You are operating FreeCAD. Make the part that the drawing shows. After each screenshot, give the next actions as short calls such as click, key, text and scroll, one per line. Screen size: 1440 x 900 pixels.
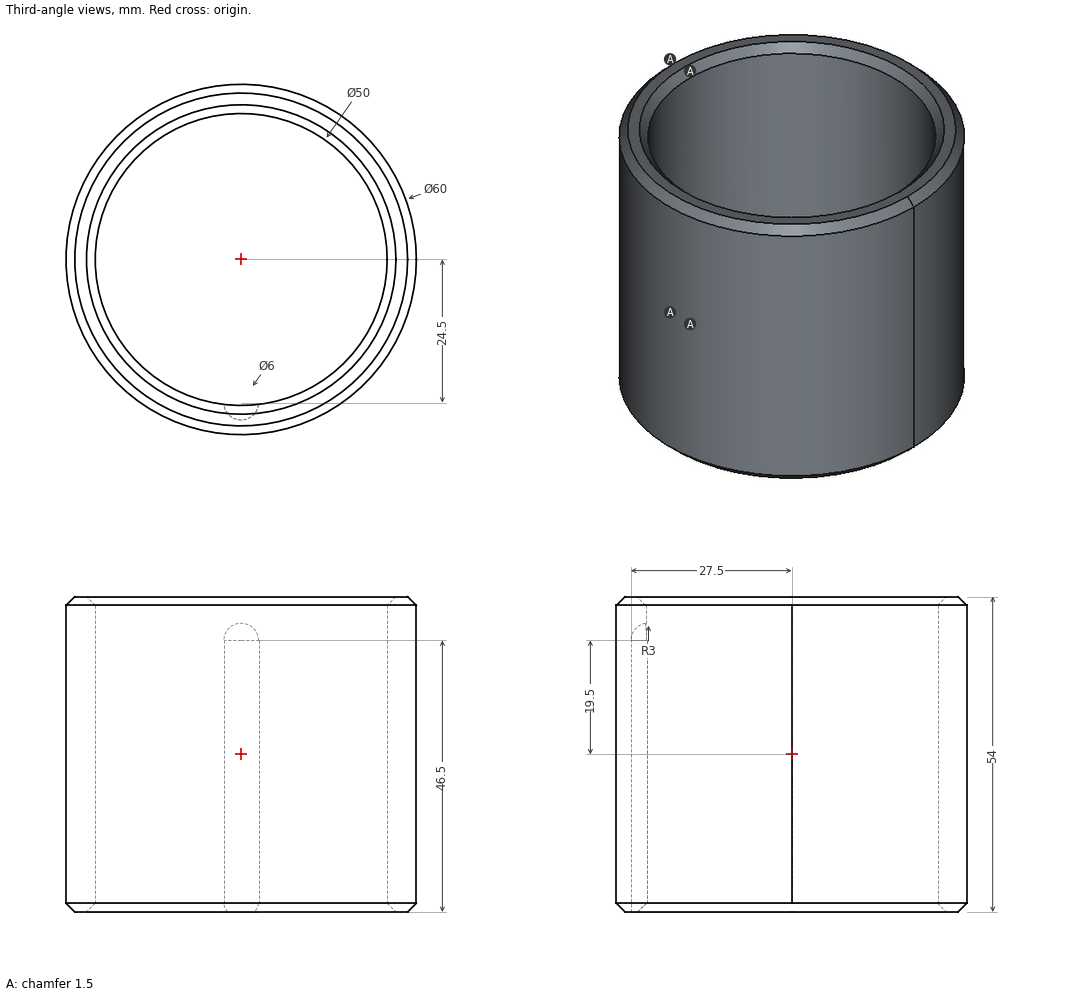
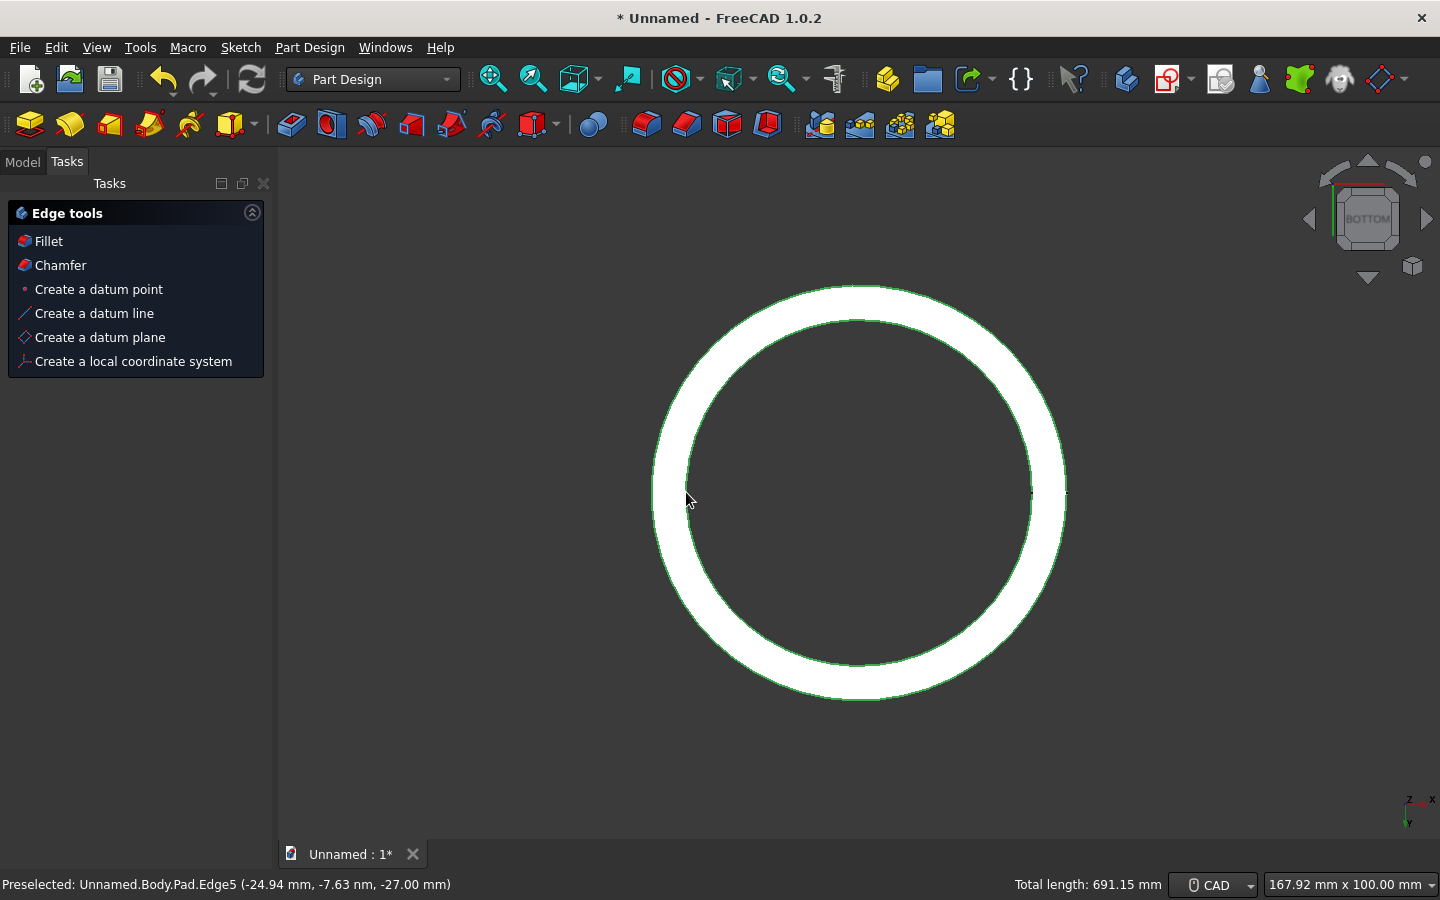
click(688, 124)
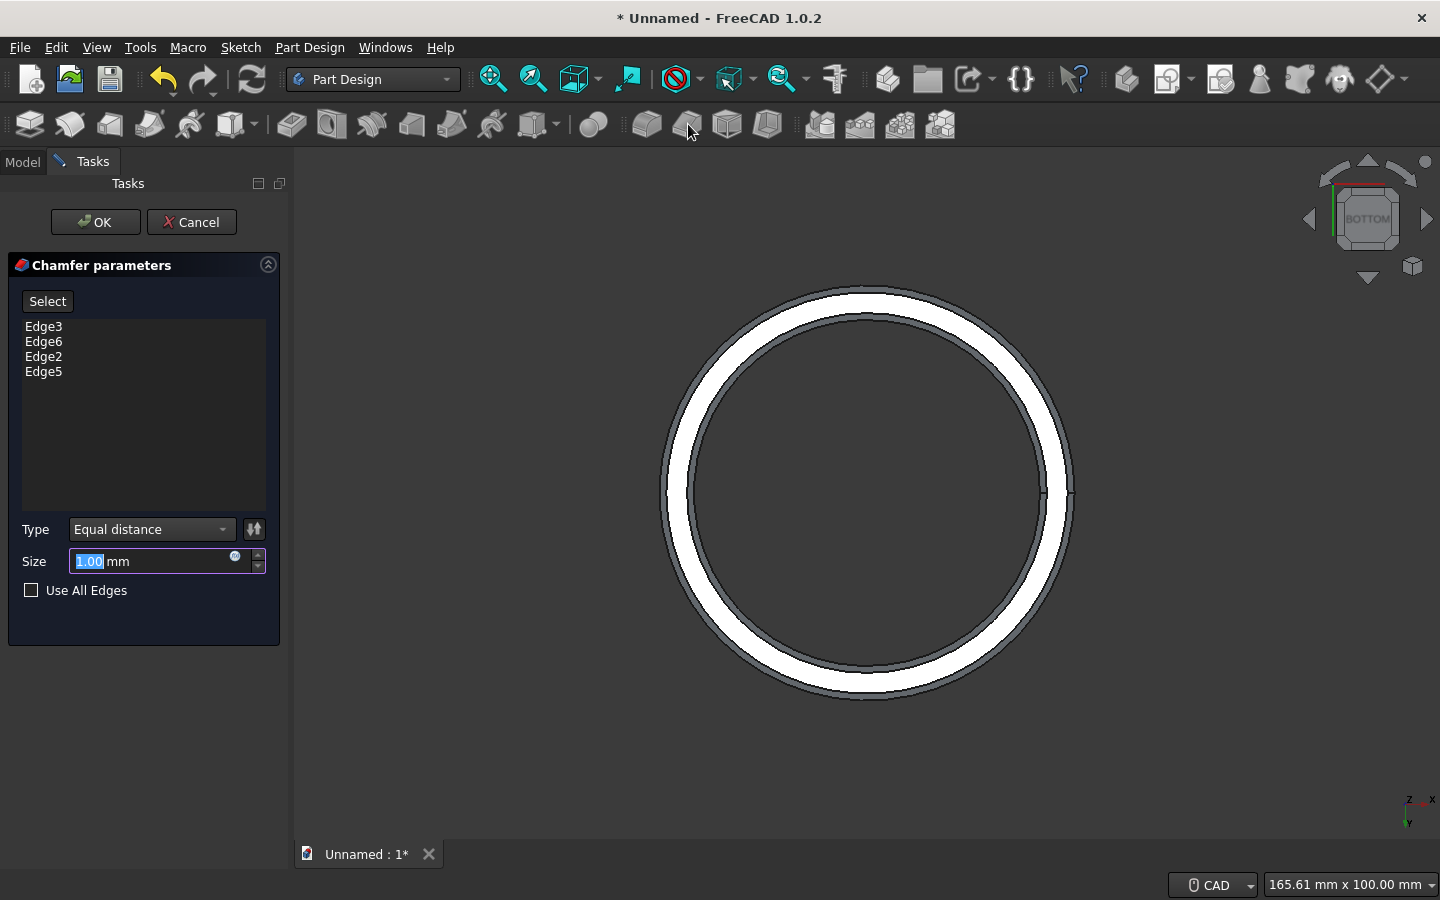
text(1.5)
key(Tab)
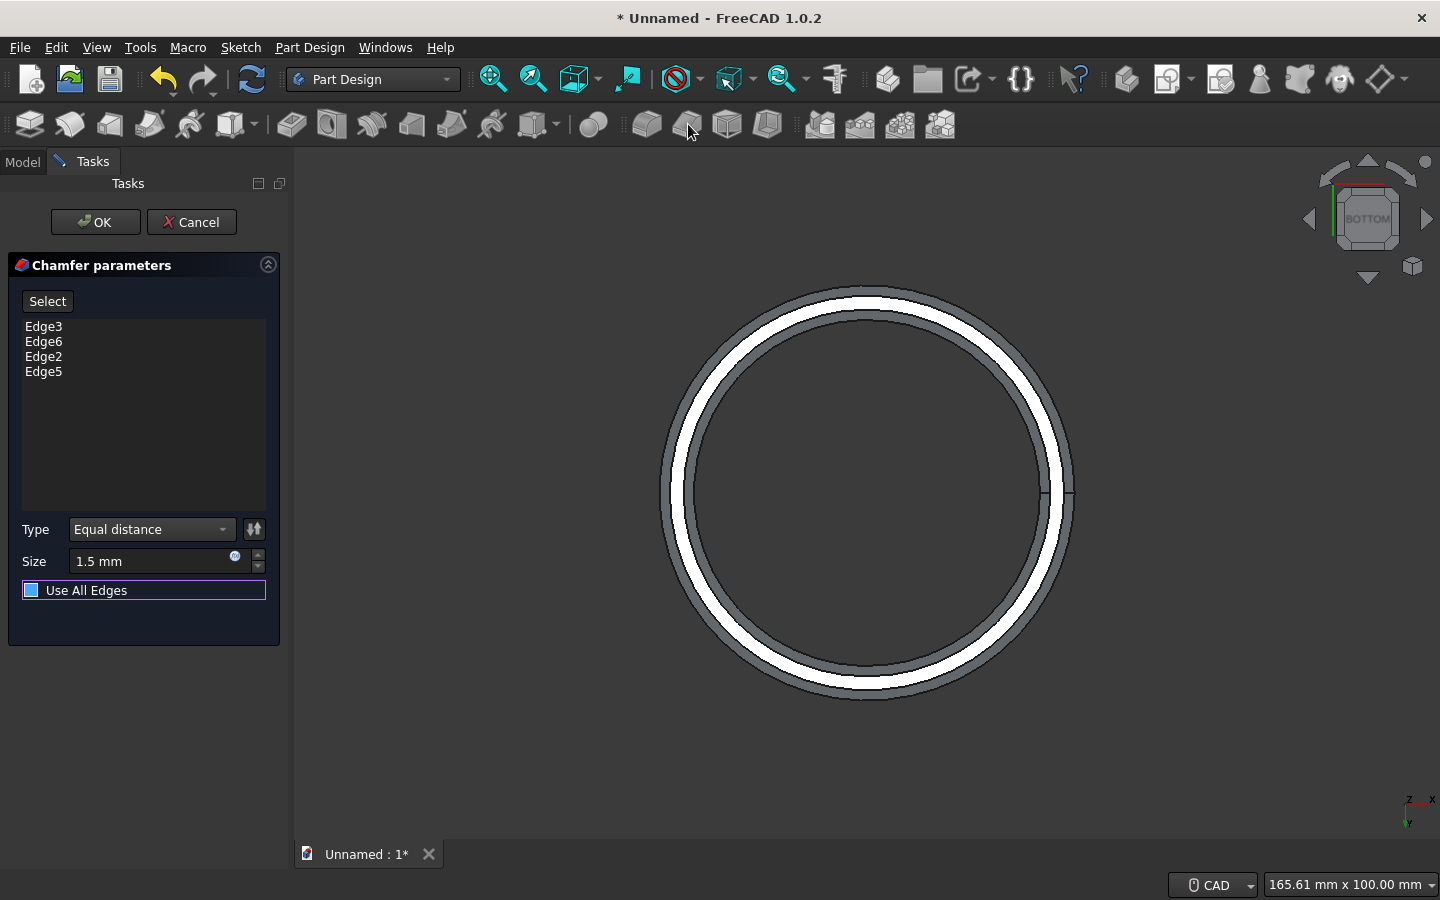
click(96, 222)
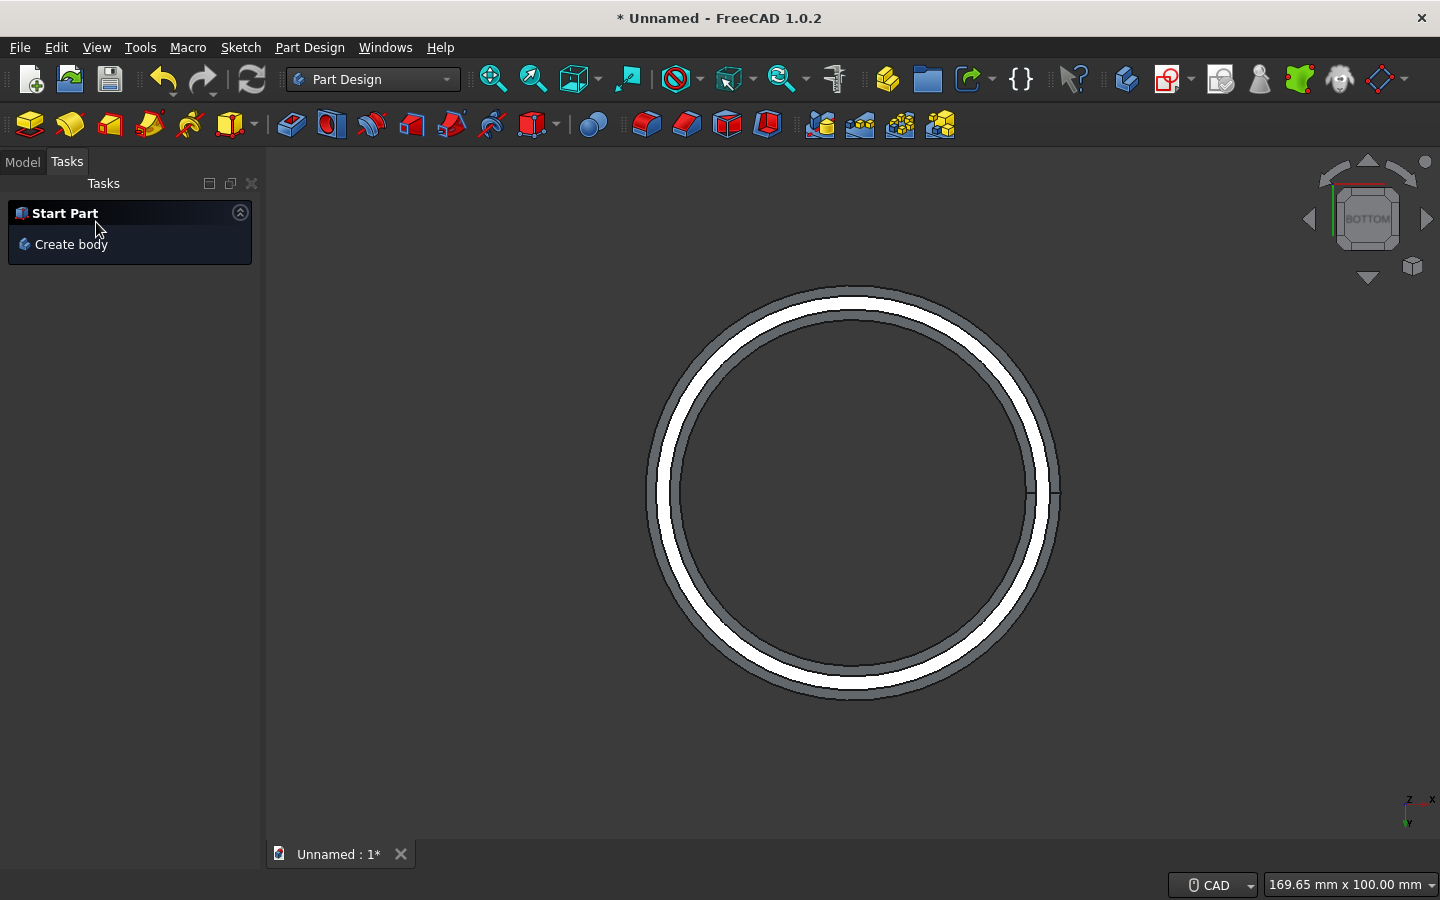
click(1168, 80)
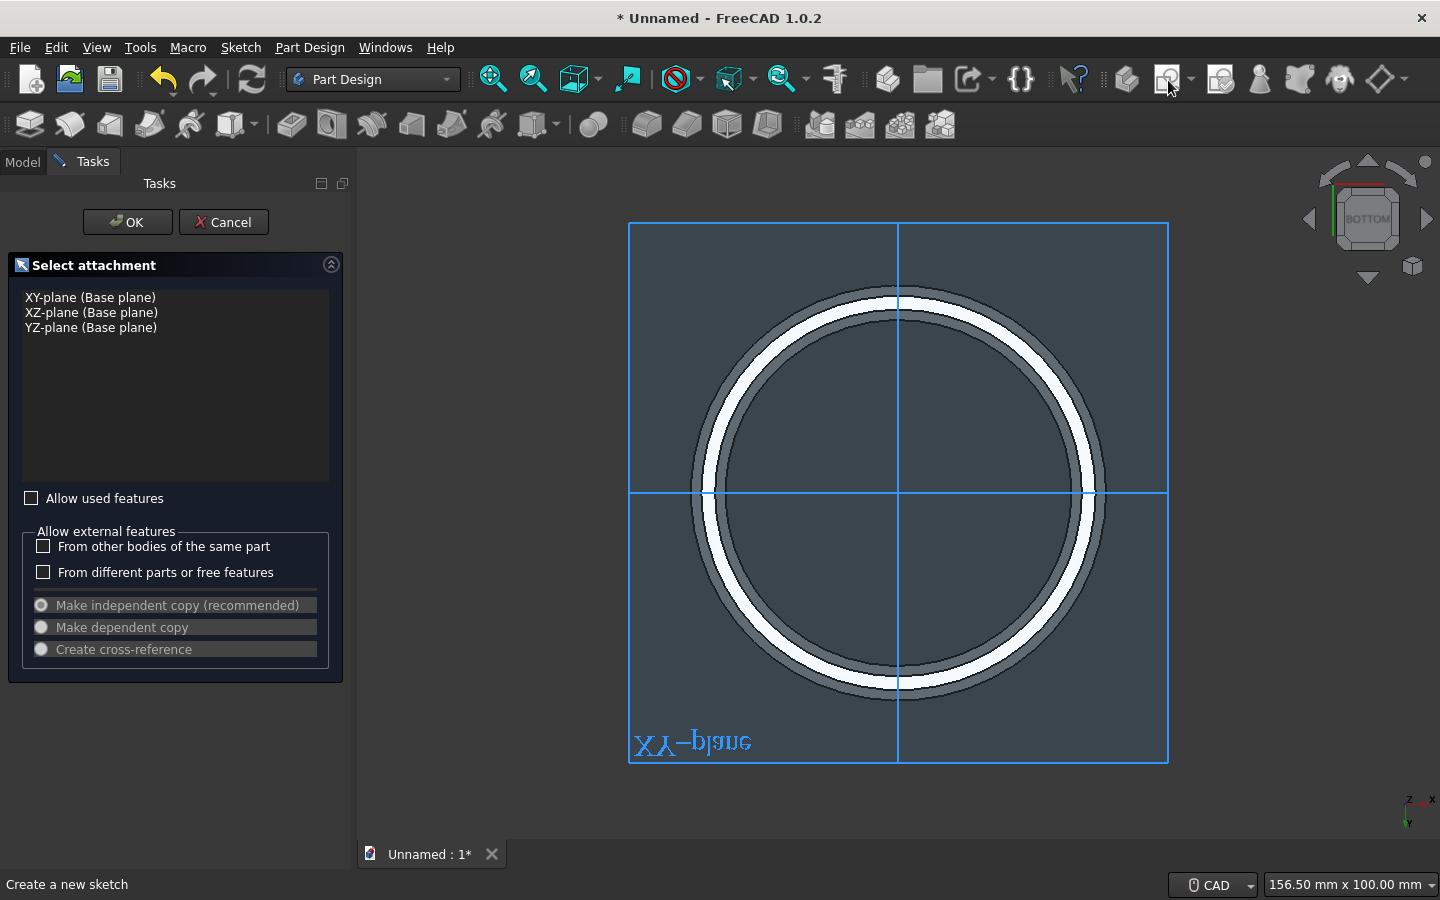
click(82, 328)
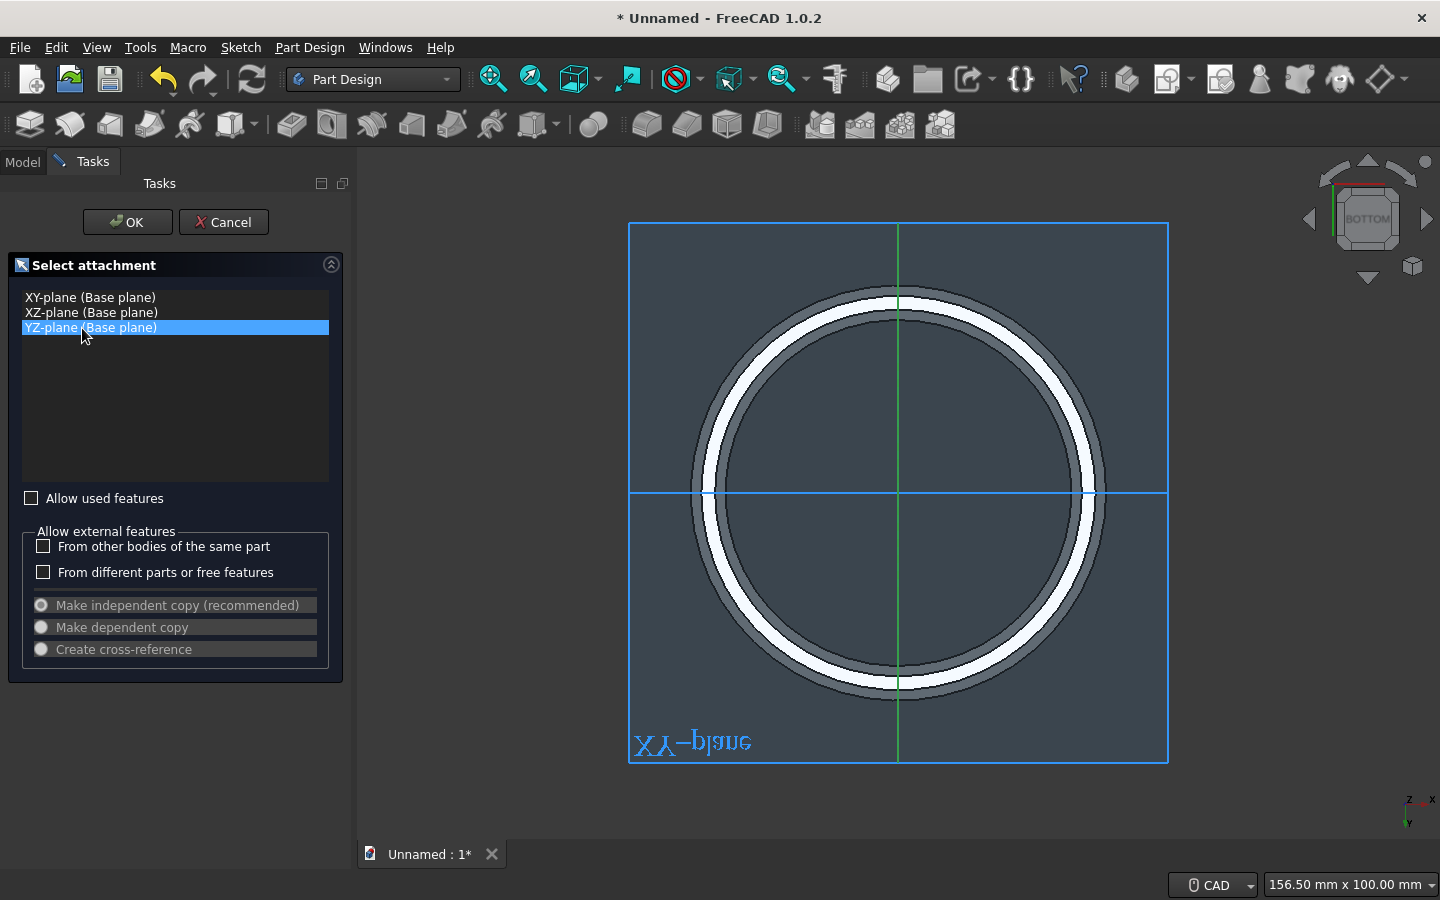
click(128, 222)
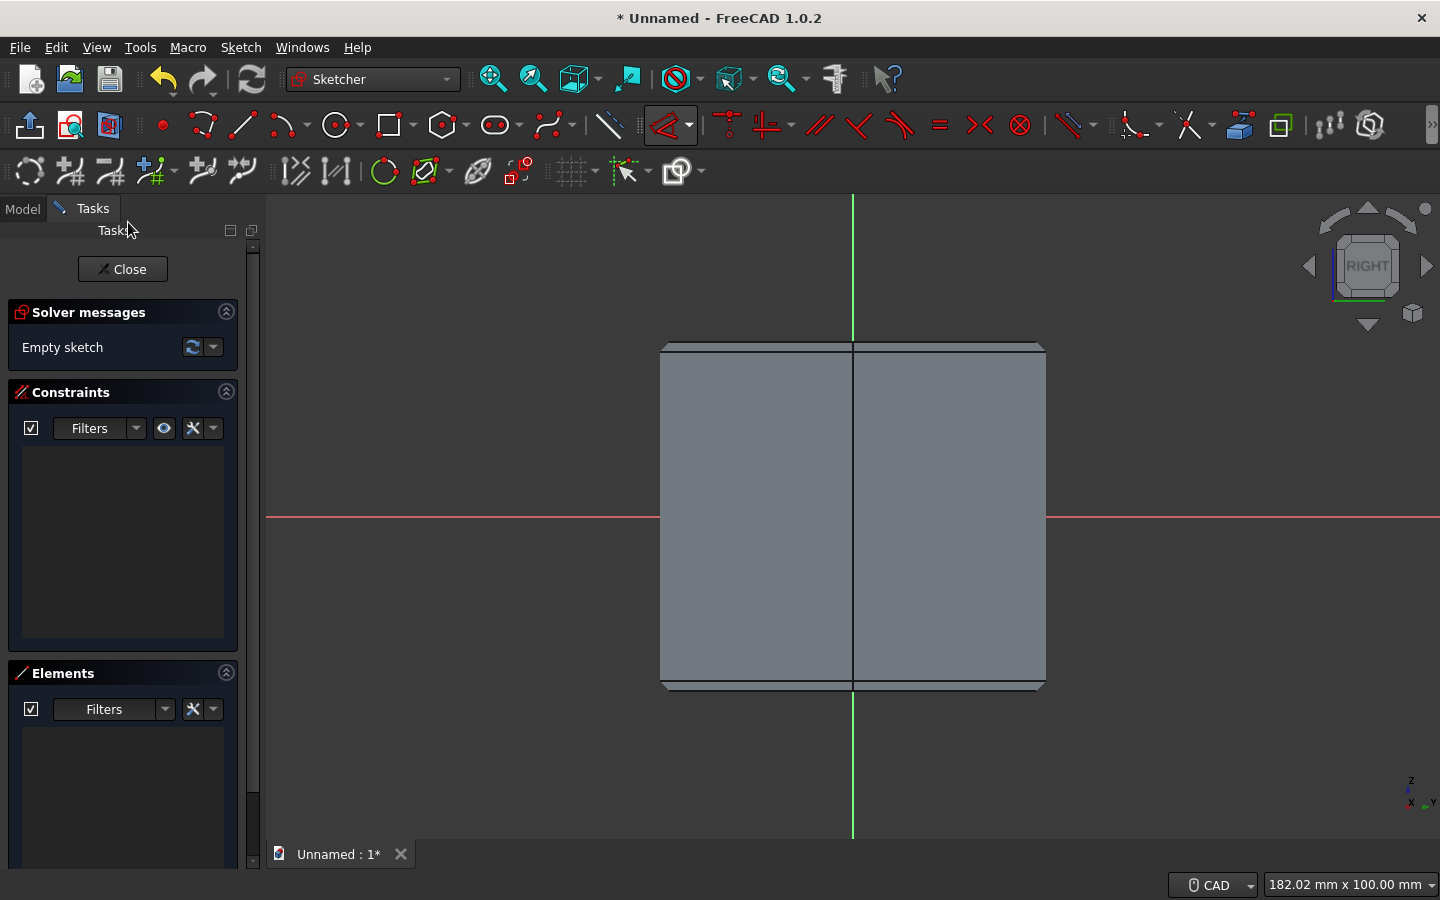
click(110, 126)